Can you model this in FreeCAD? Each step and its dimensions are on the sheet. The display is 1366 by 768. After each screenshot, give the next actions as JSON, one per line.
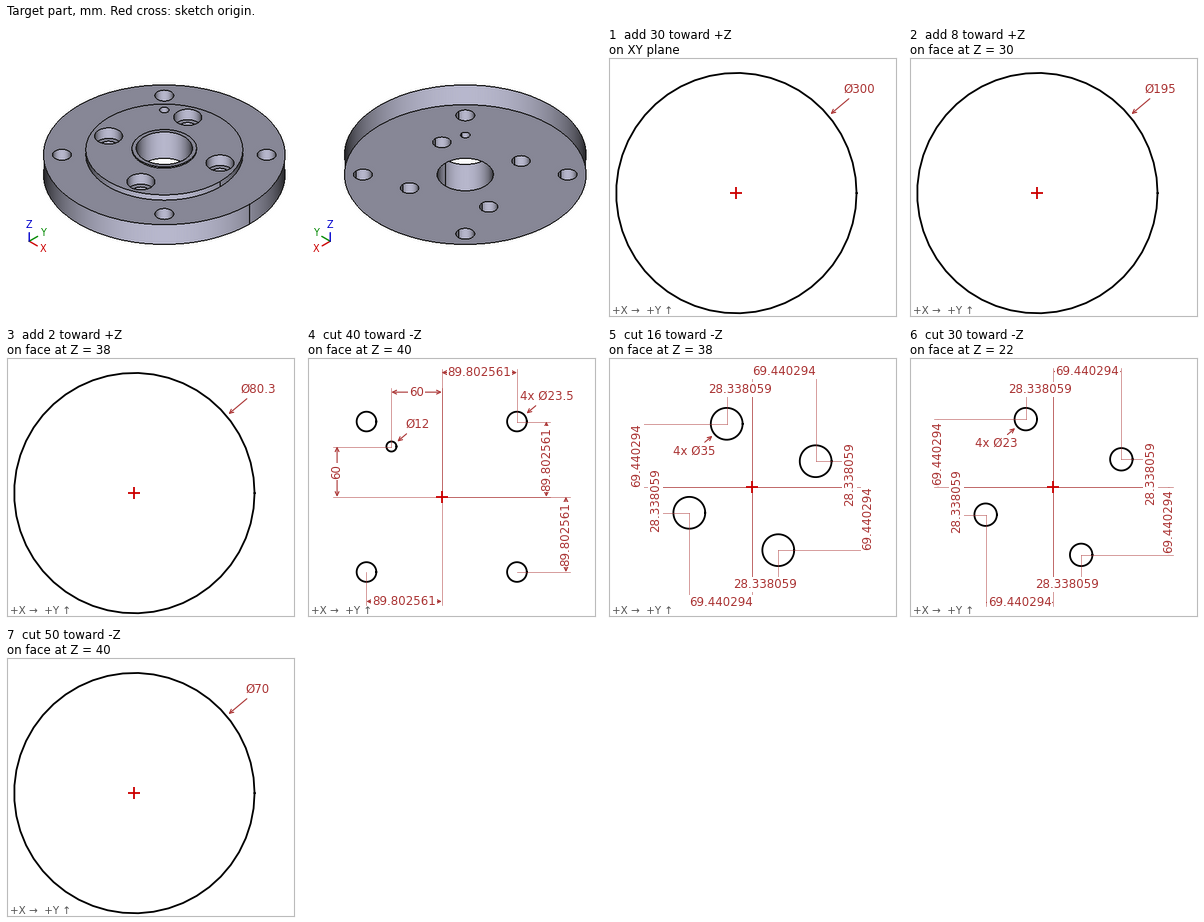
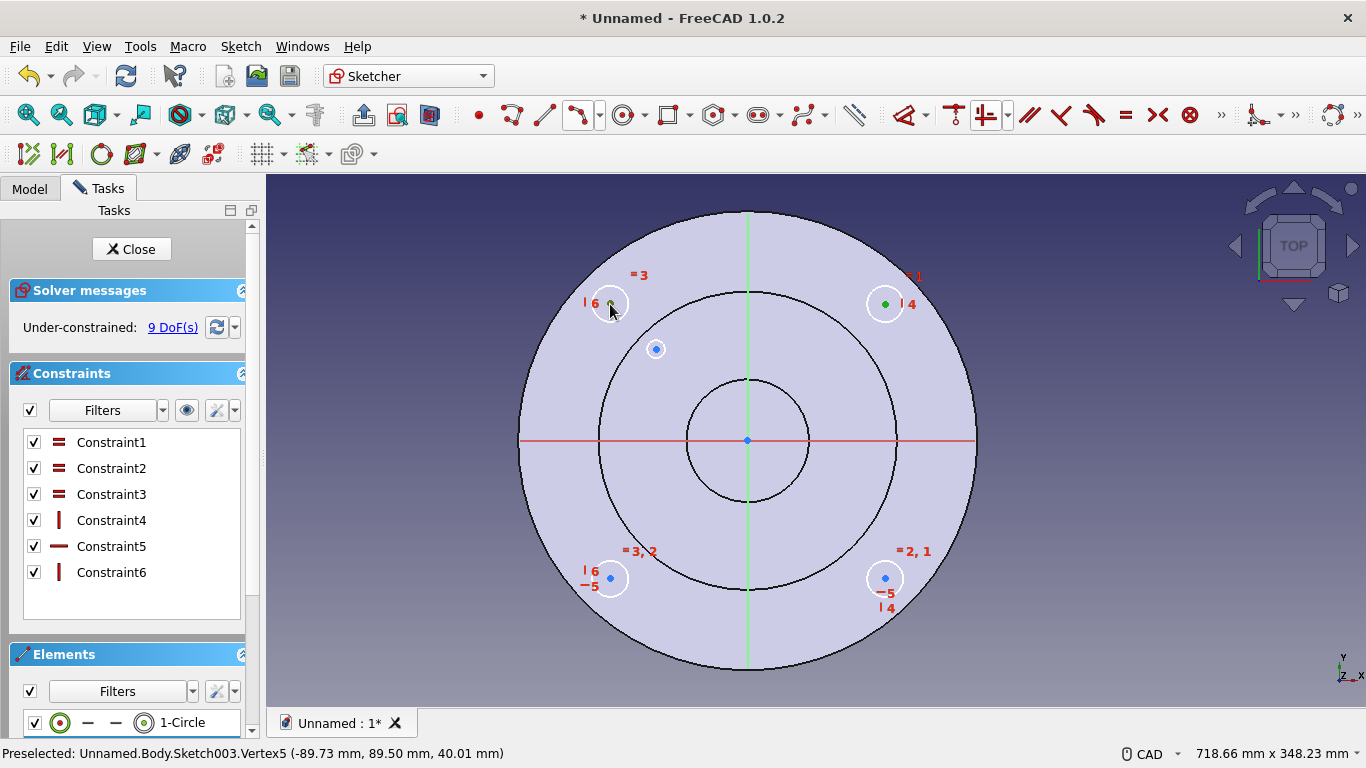
{"action": "left_click", "coordinate": [1008, 116]}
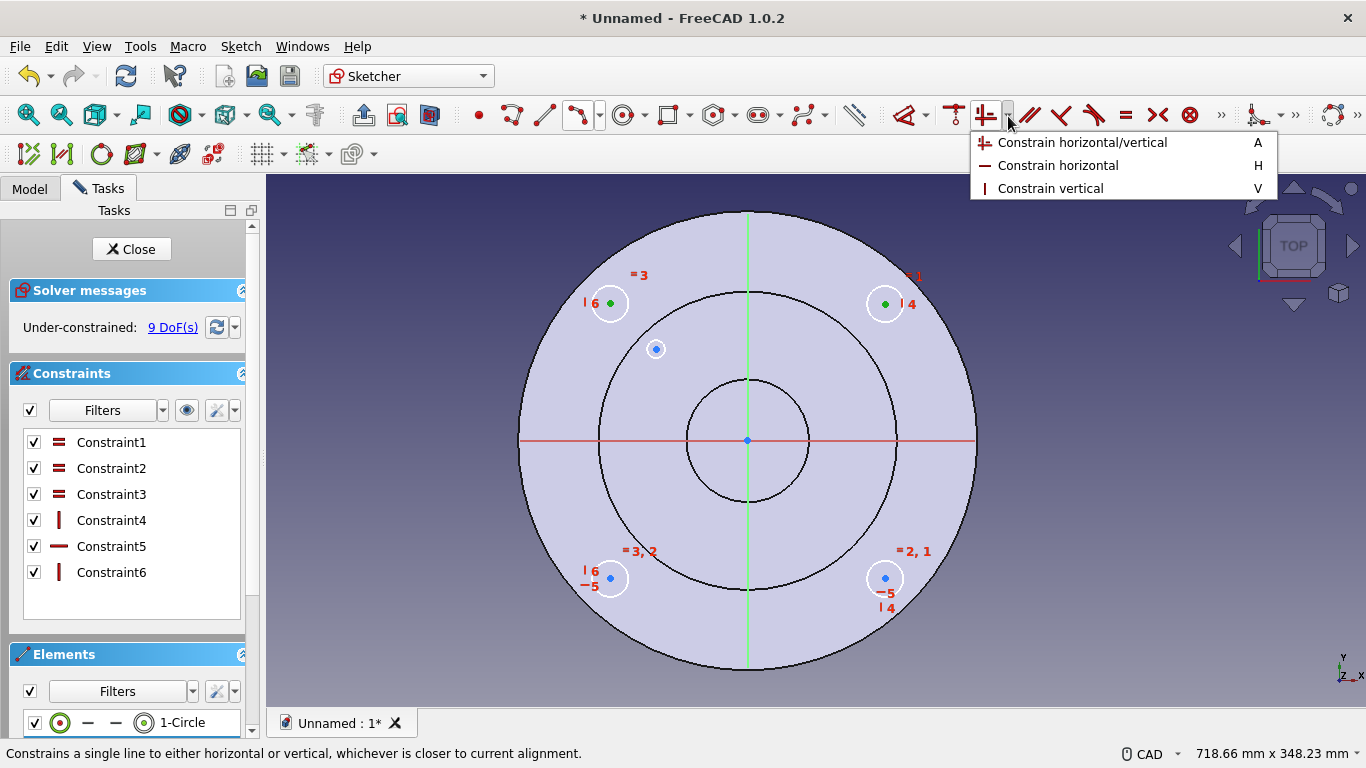
{"action": "left_click", "coordinate": [1124, 166]}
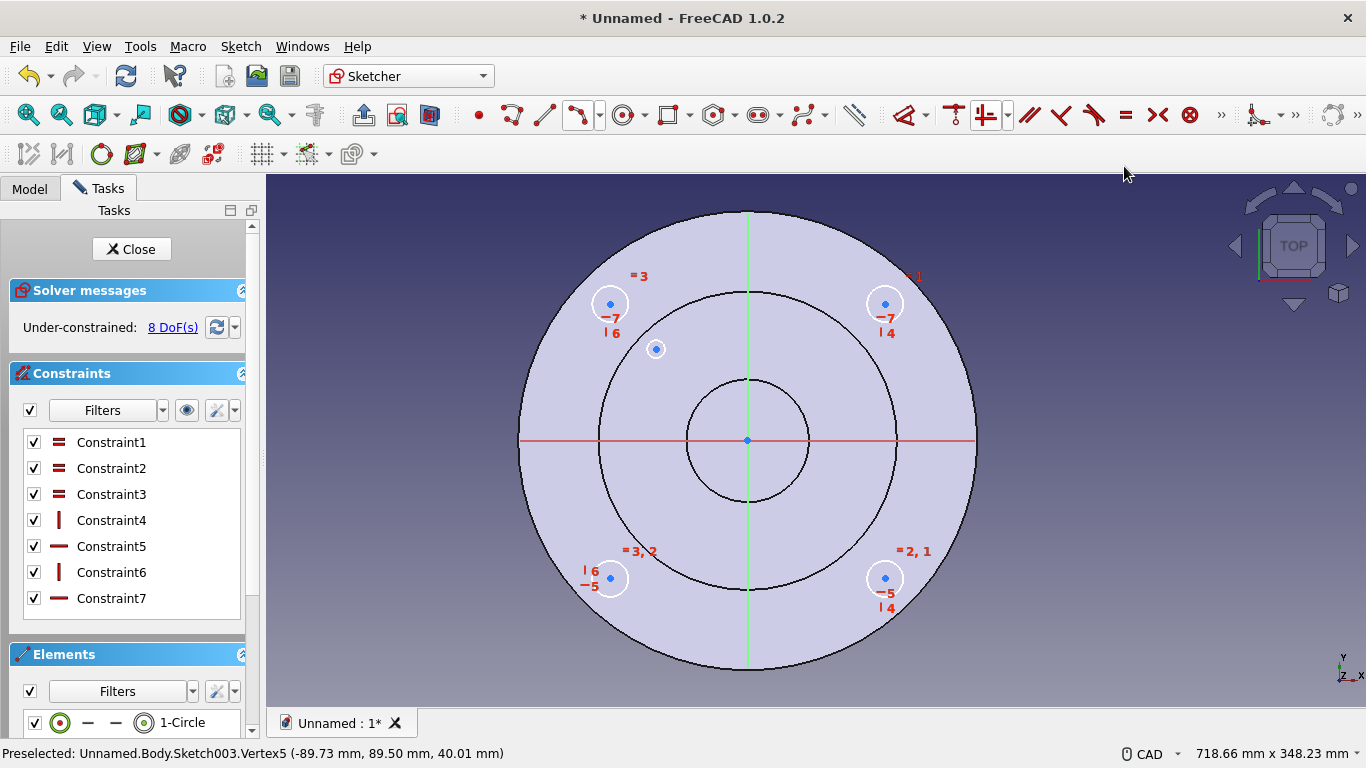
{"action": "left_click", "coordinate": [904, 116]}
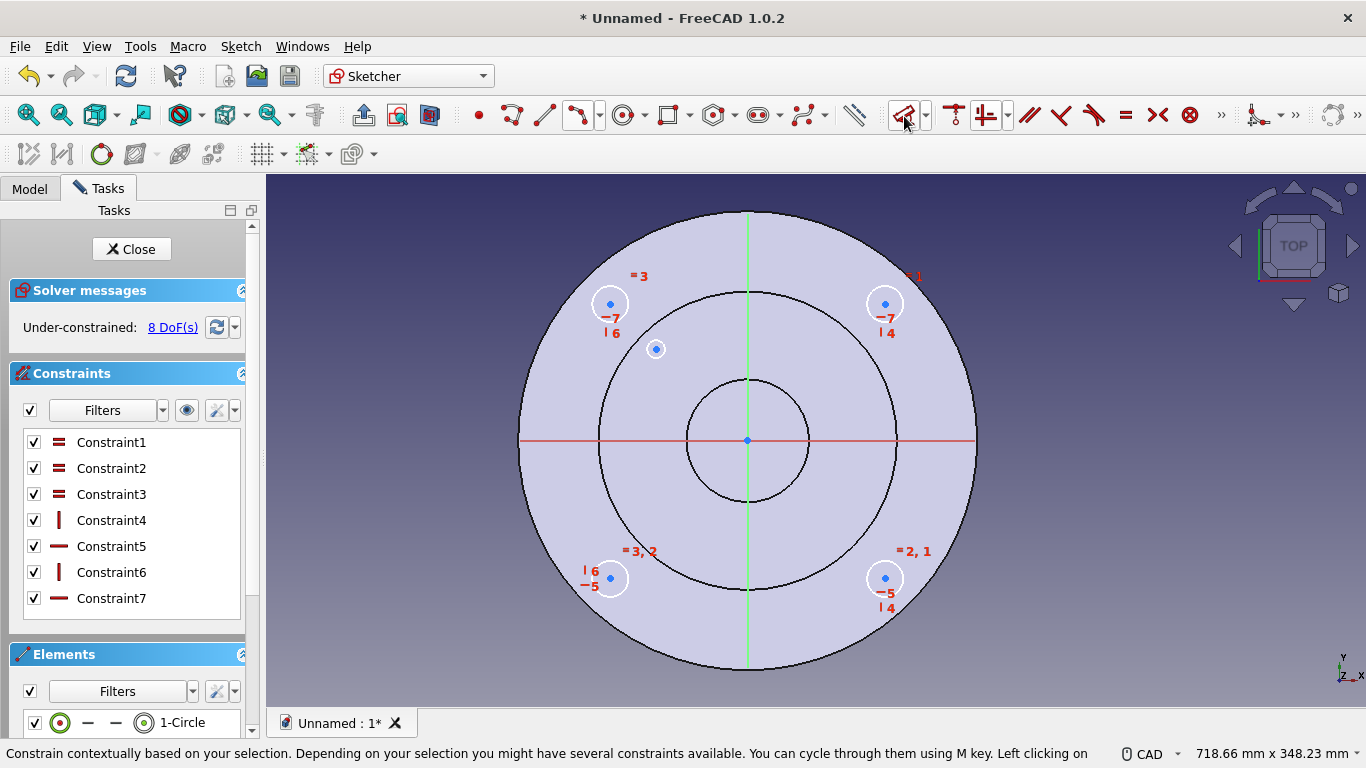
{"action": "scroll", "coordinate": [662, 355], "scroll_direction": "up", "scroll_amount": 4}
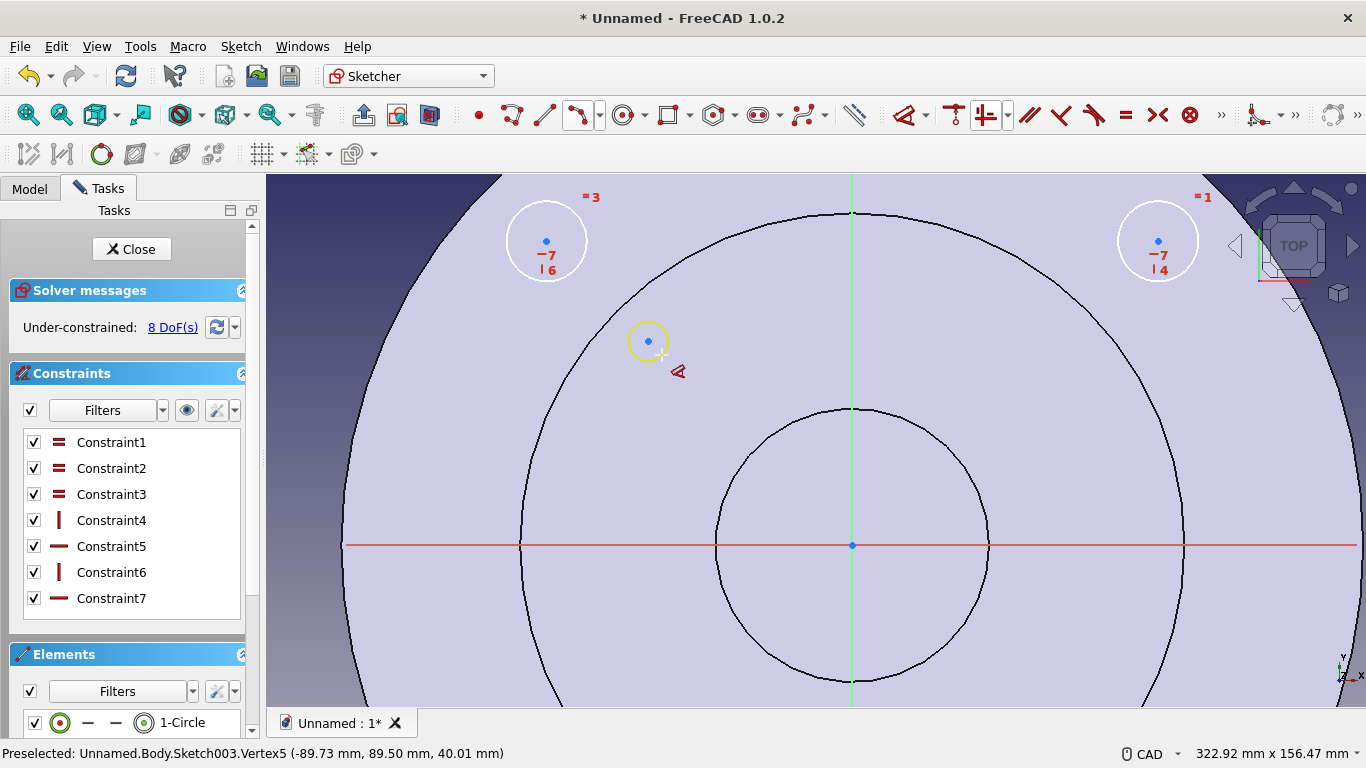
{"action": "left_click", "coordinate": [662, 355]}
{"action": "left_click", "coordinate": [685, 377]}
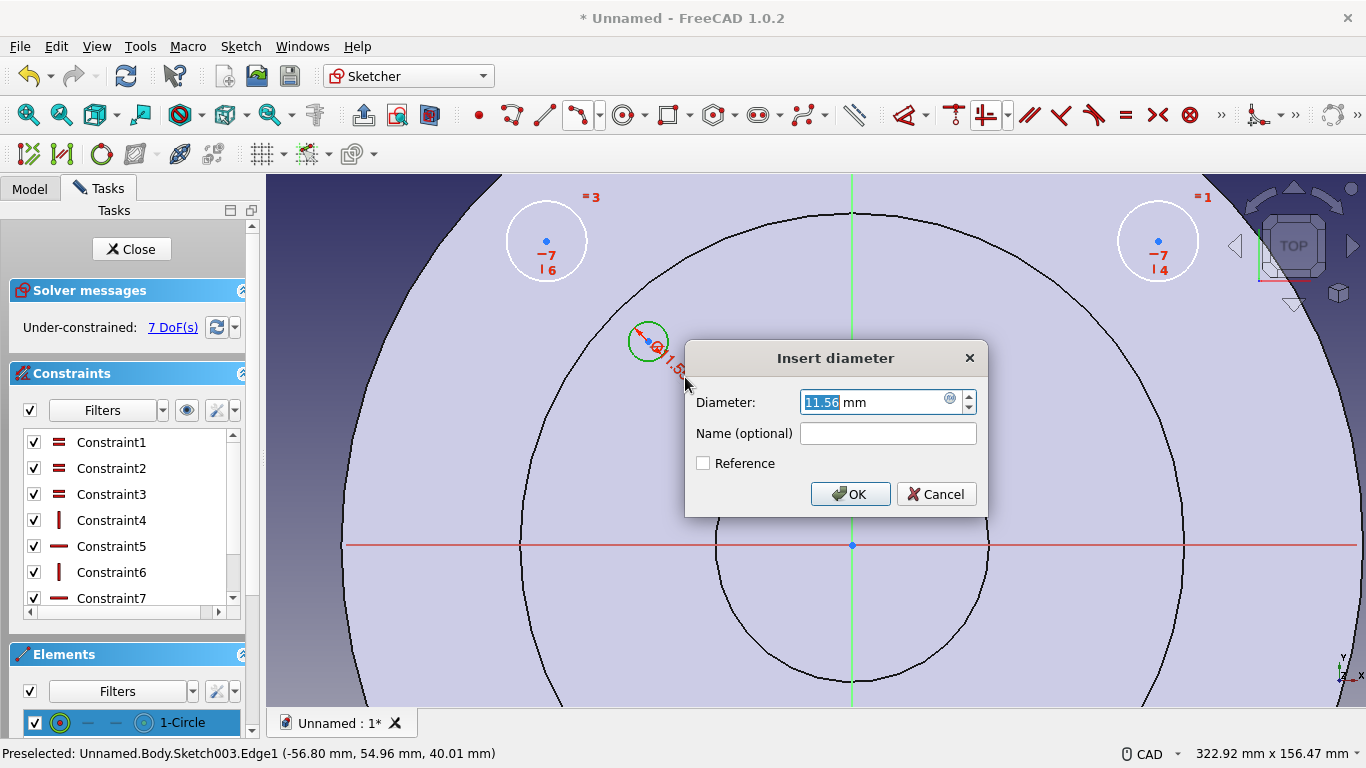
{"action": "type", "text": "12"}
{"action": "key", "text": "Return"}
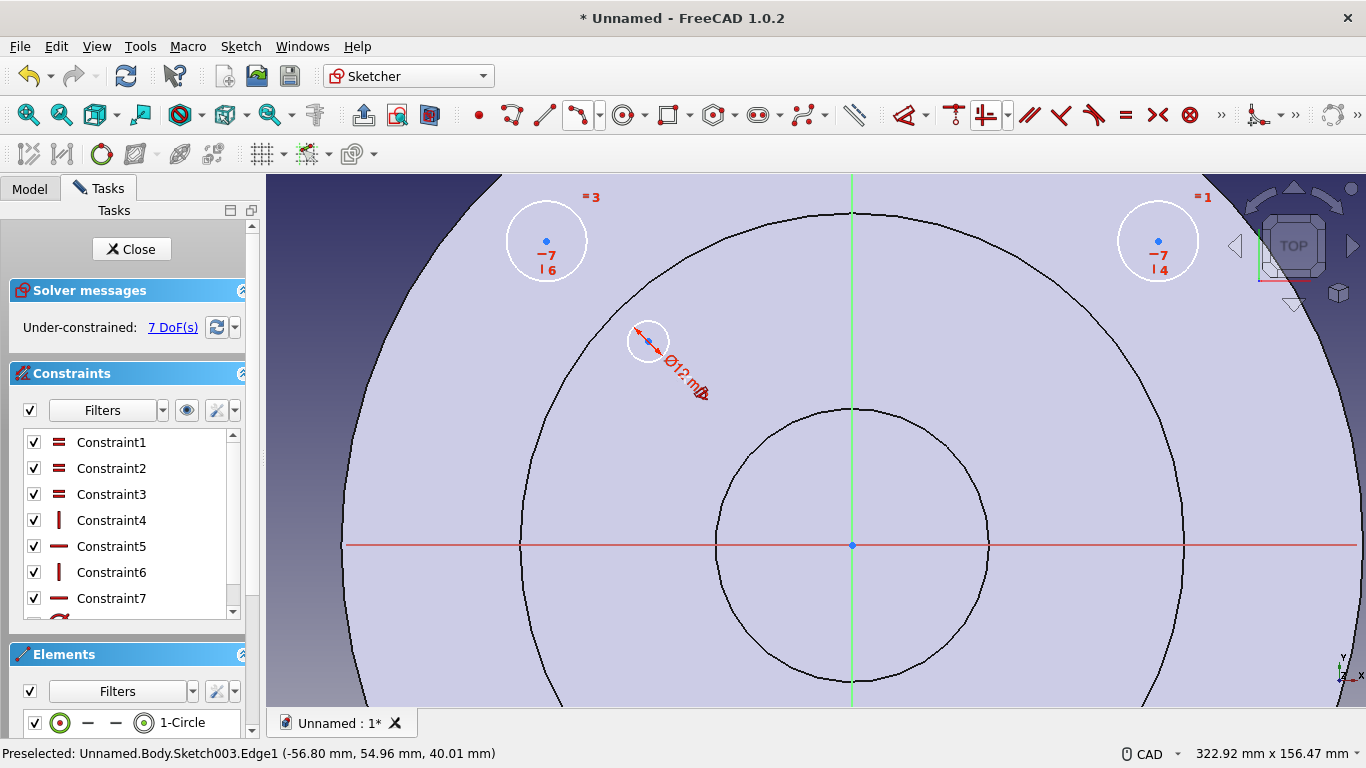
{"action": "left_click", "coordinate": [1187, 213]}
{"action": "left_click", "coordinate": [1107, 292]}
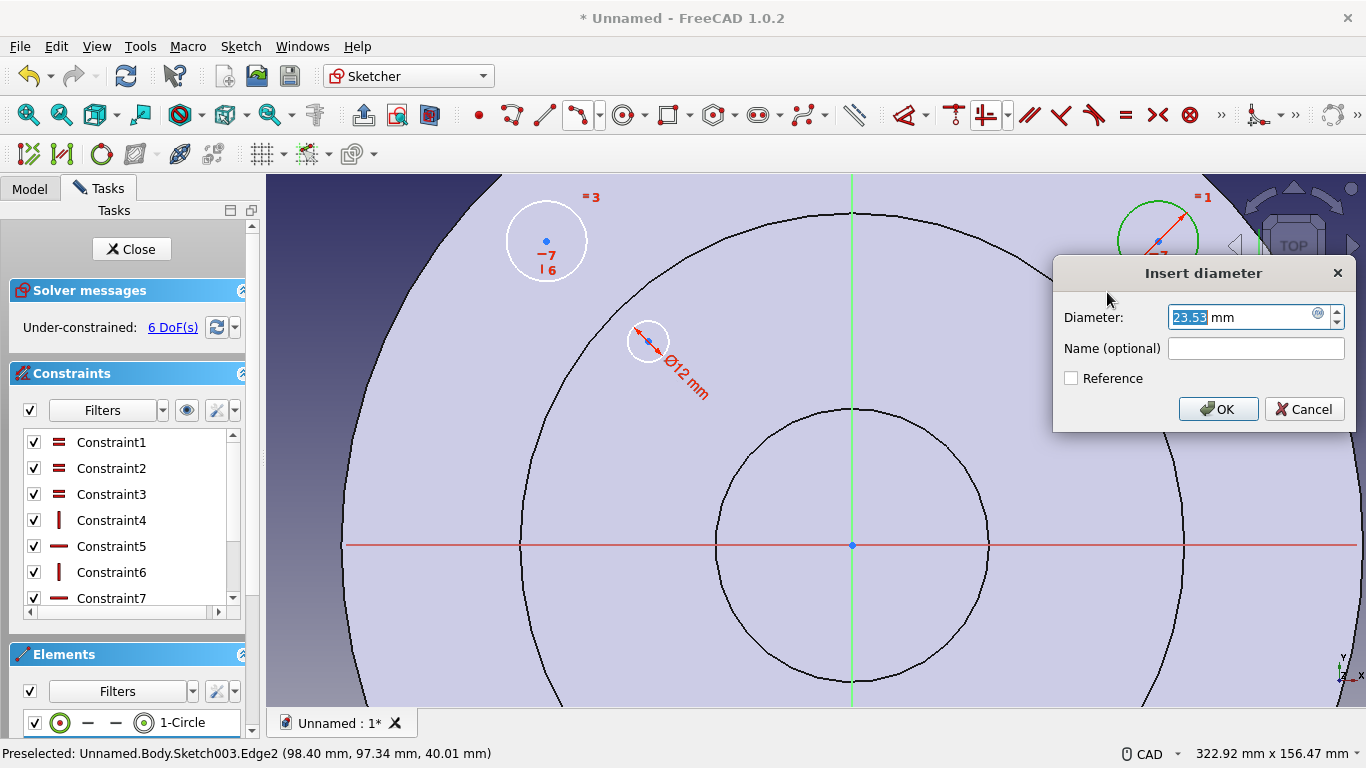
{"action": "type", "text": "23.5"}
{"action": "key", "text": "Return"}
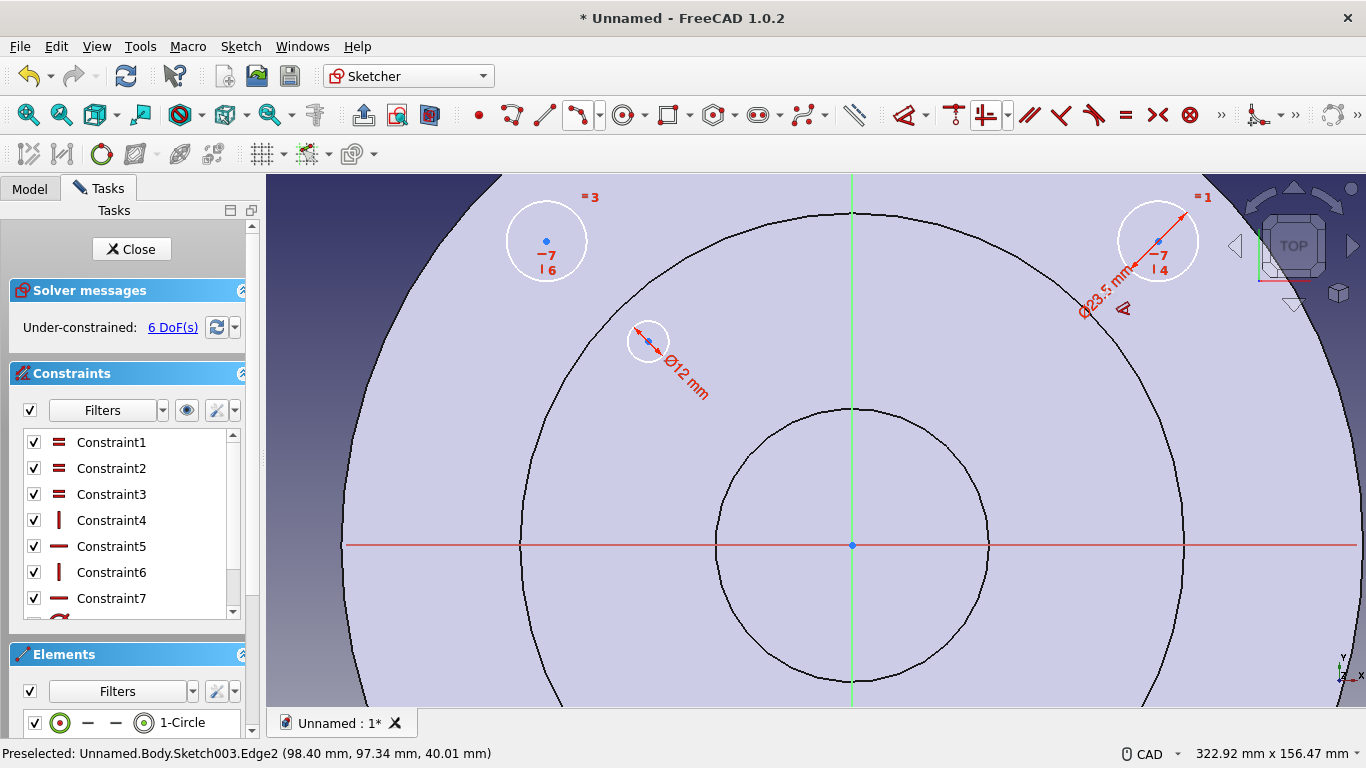
{"action": "left_click", "coordinate": [648, 342]}
{"action": "left_click", "coordinate": [750, 308]}